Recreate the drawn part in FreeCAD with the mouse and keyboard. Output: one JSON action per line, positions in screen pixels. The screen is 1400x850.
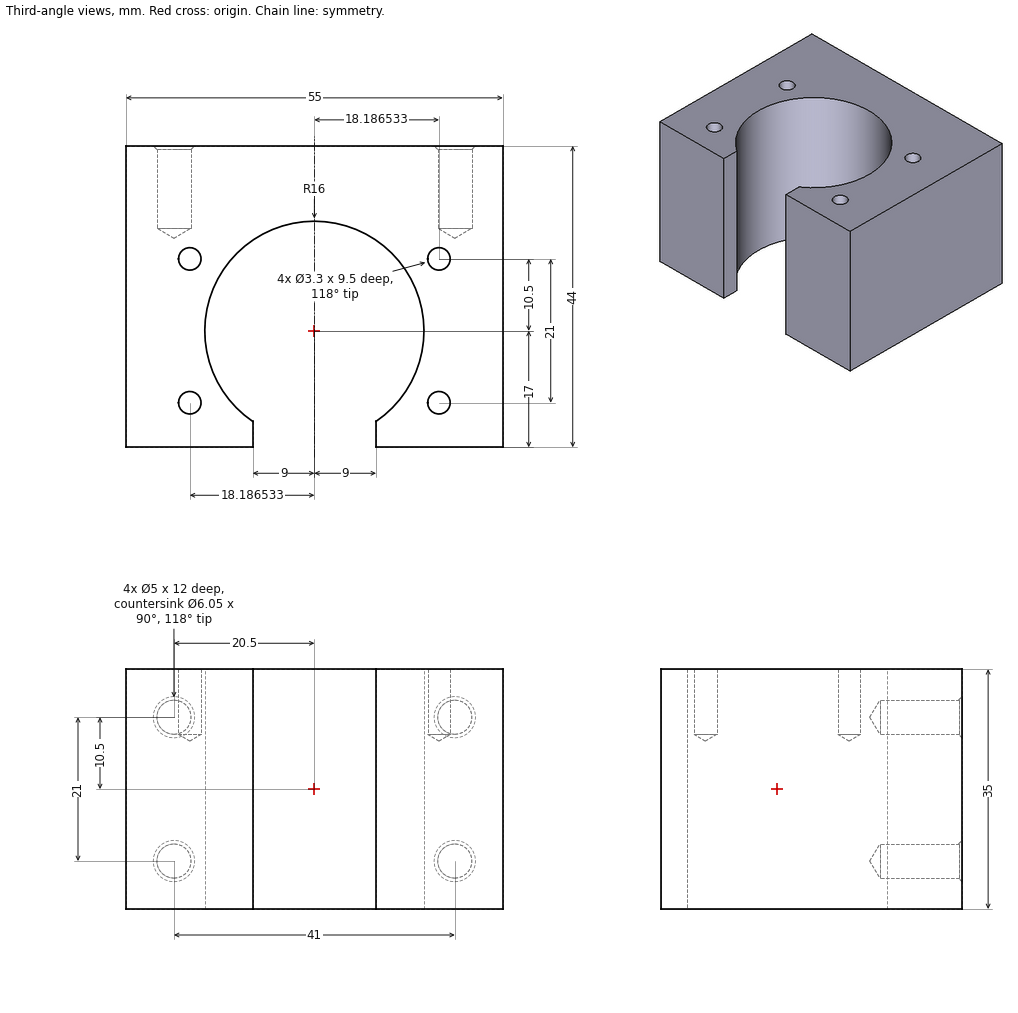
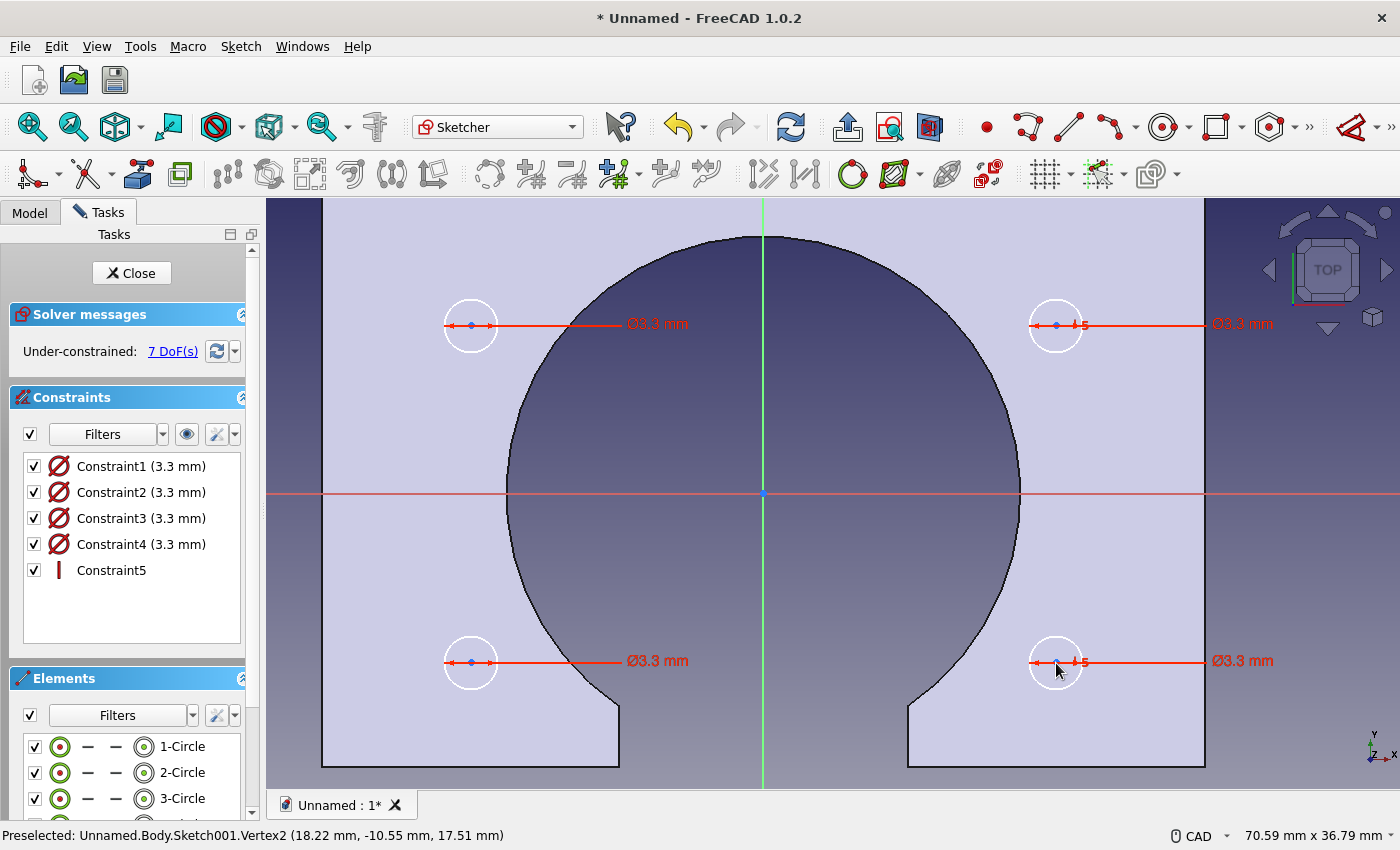
{"action": "left_click", "coordinate": [1056, 663]}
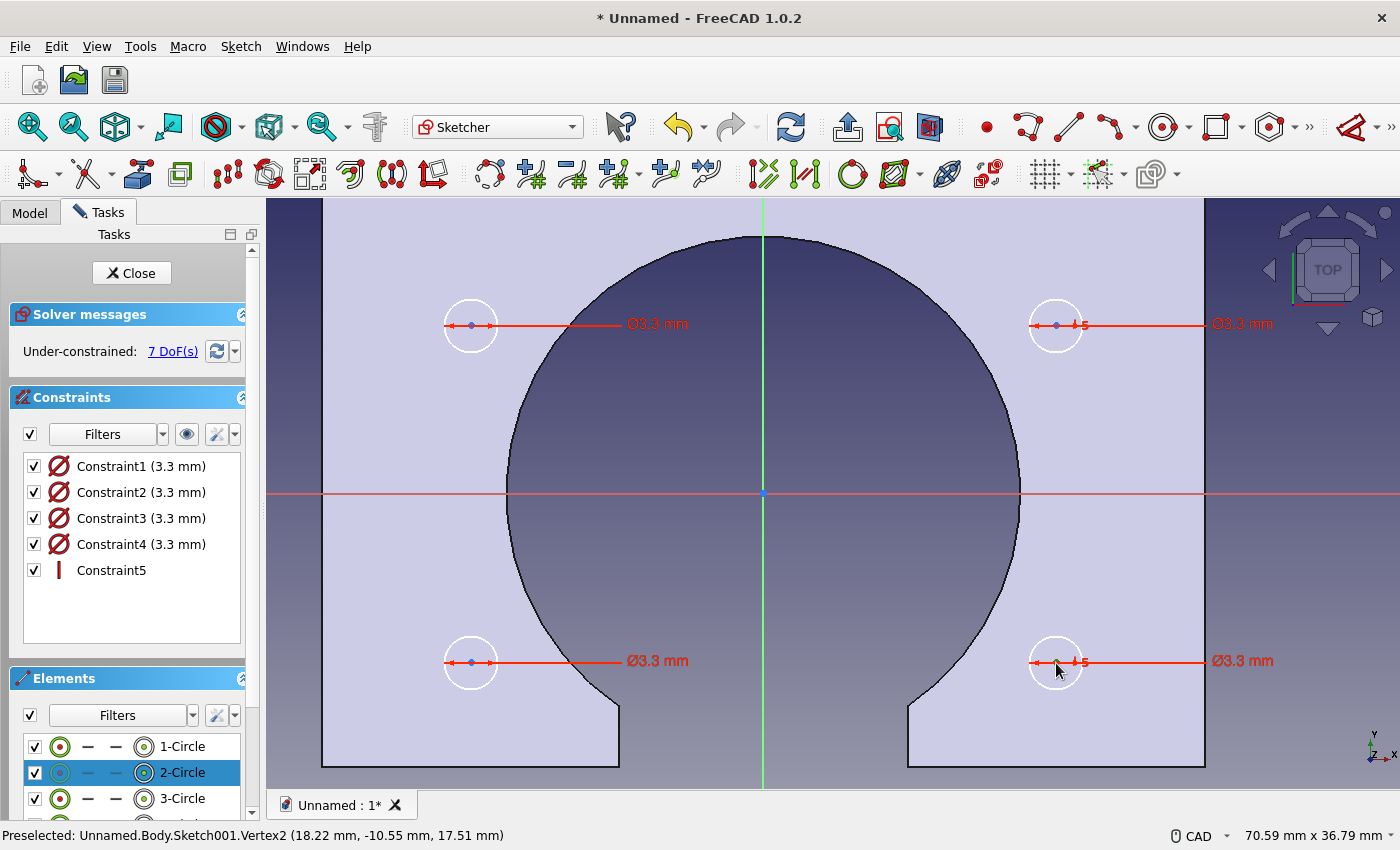
{"action": "left_click", "coordinate": [471, 663]}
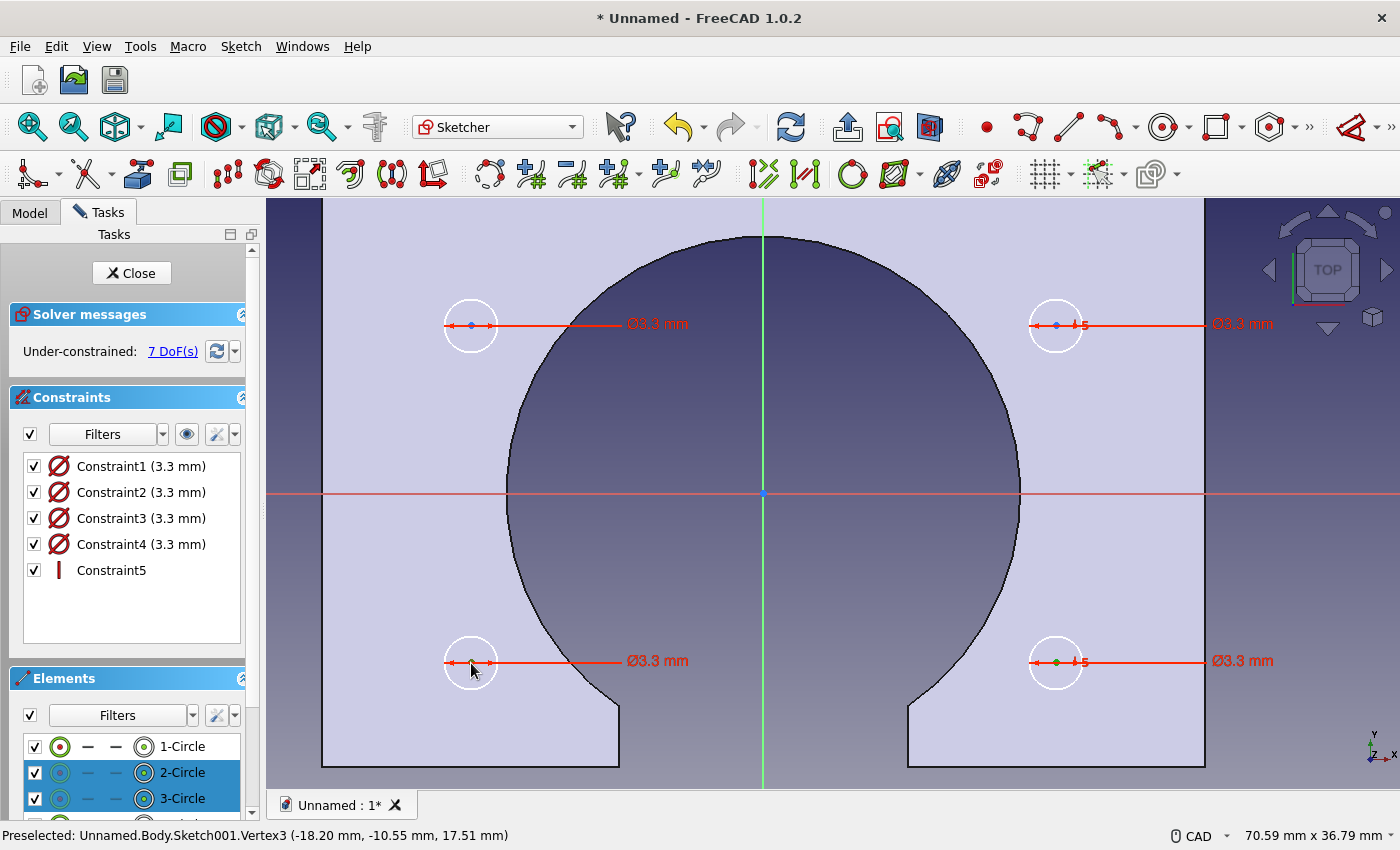
{"action": "key", "text": "h"}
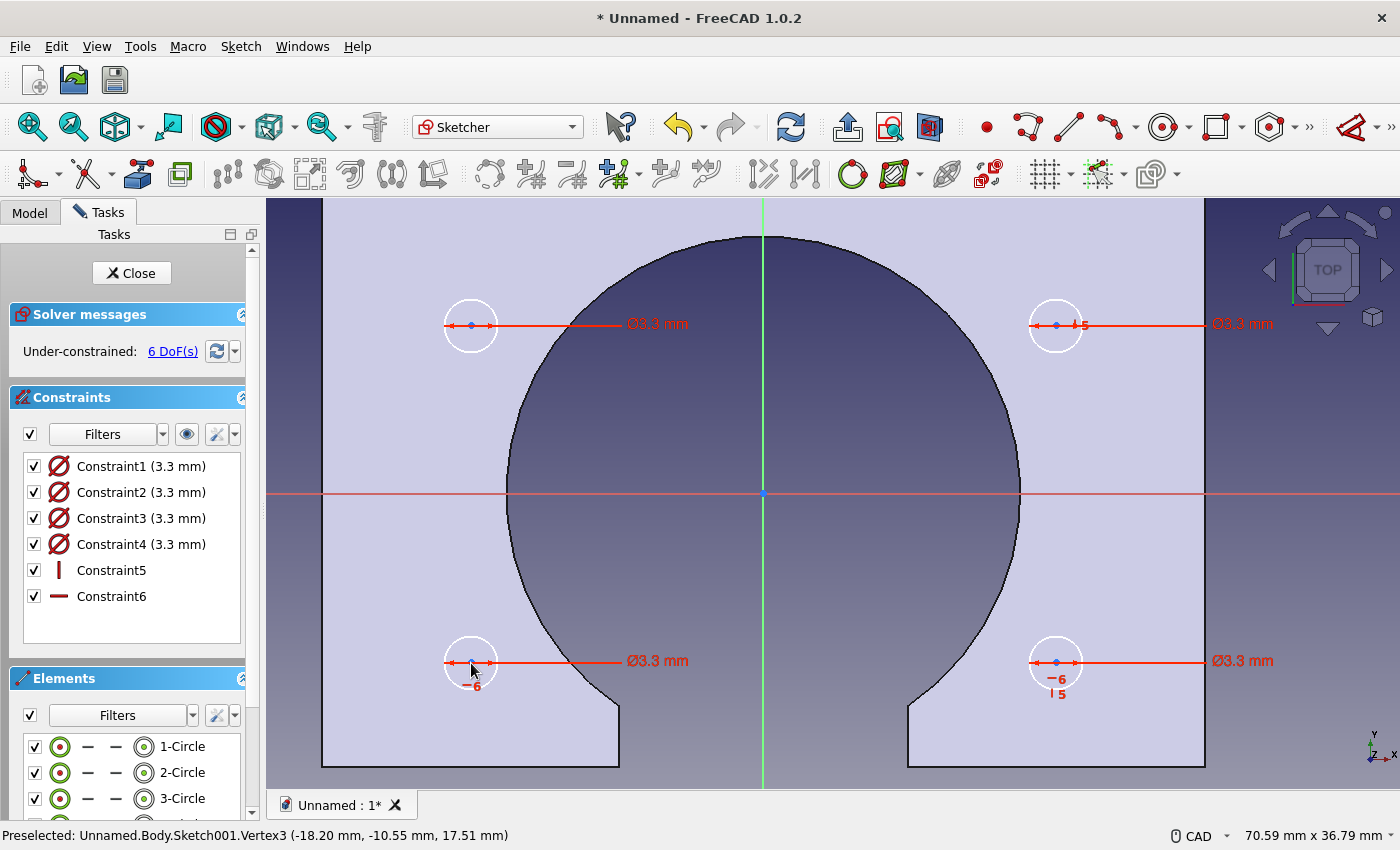
{"action": "left_click", "coordinate": [471, 663]}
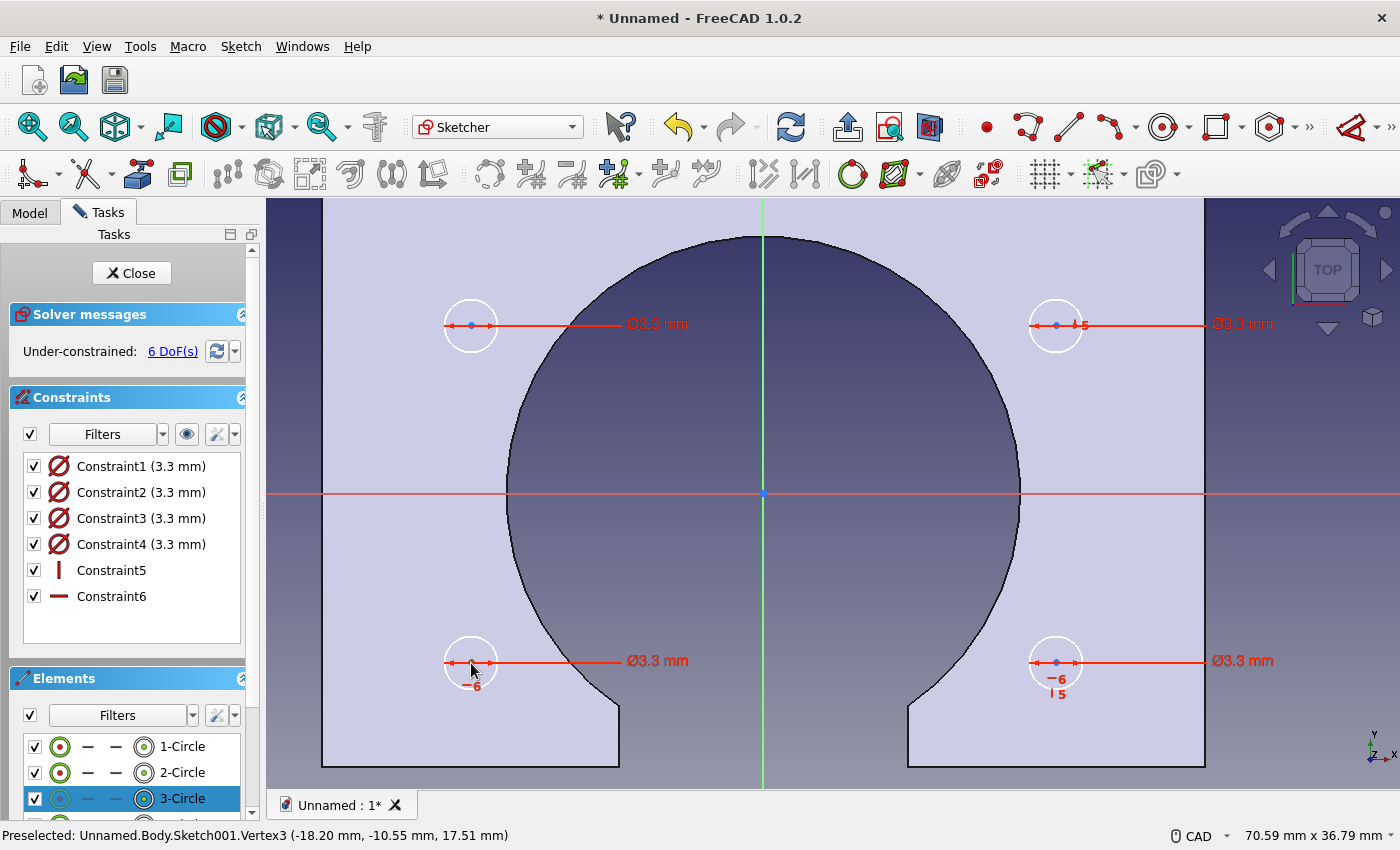
{"action": "left_click", "coordinate": [471, 326]}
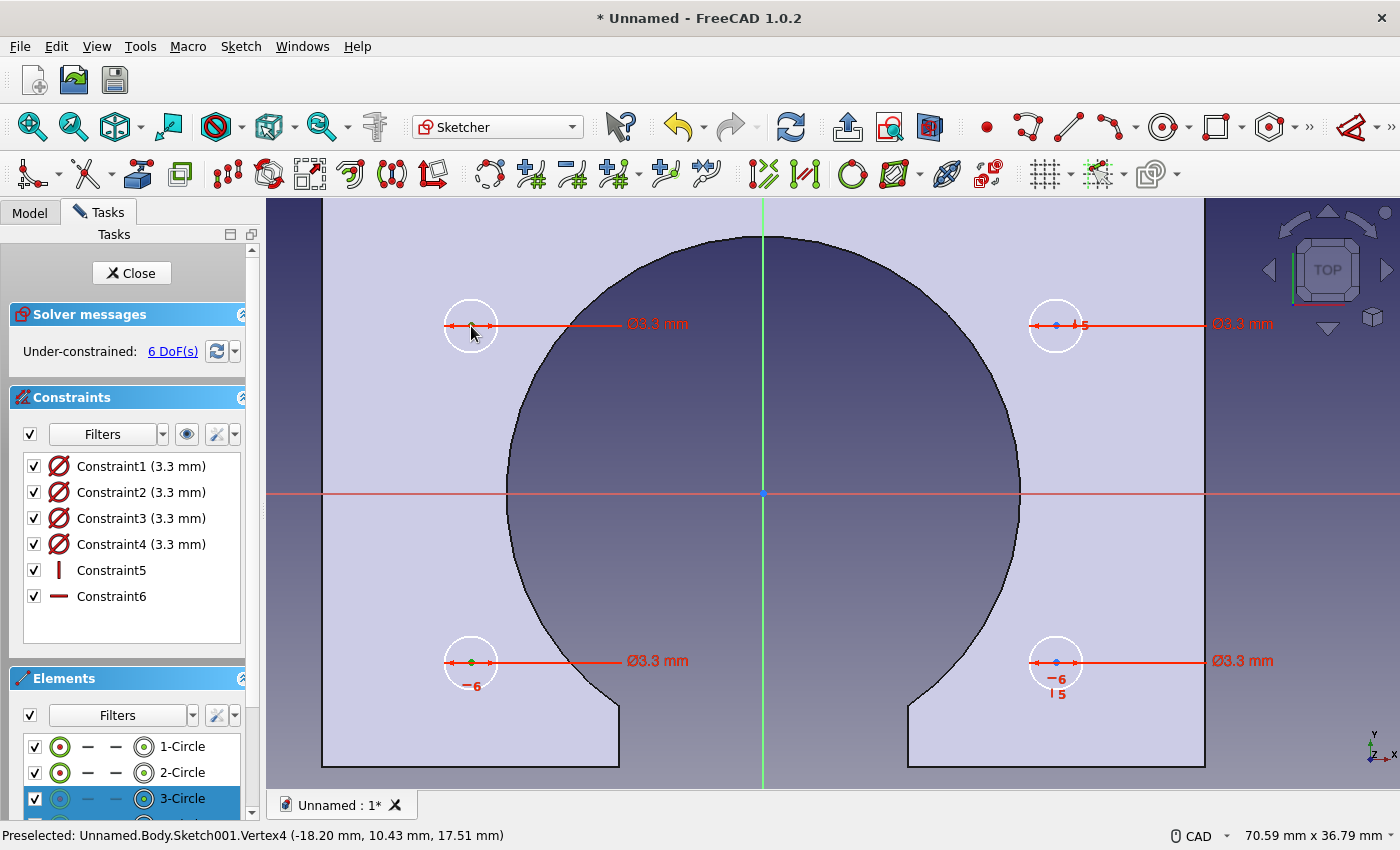
{"action": "key", "text": "v"}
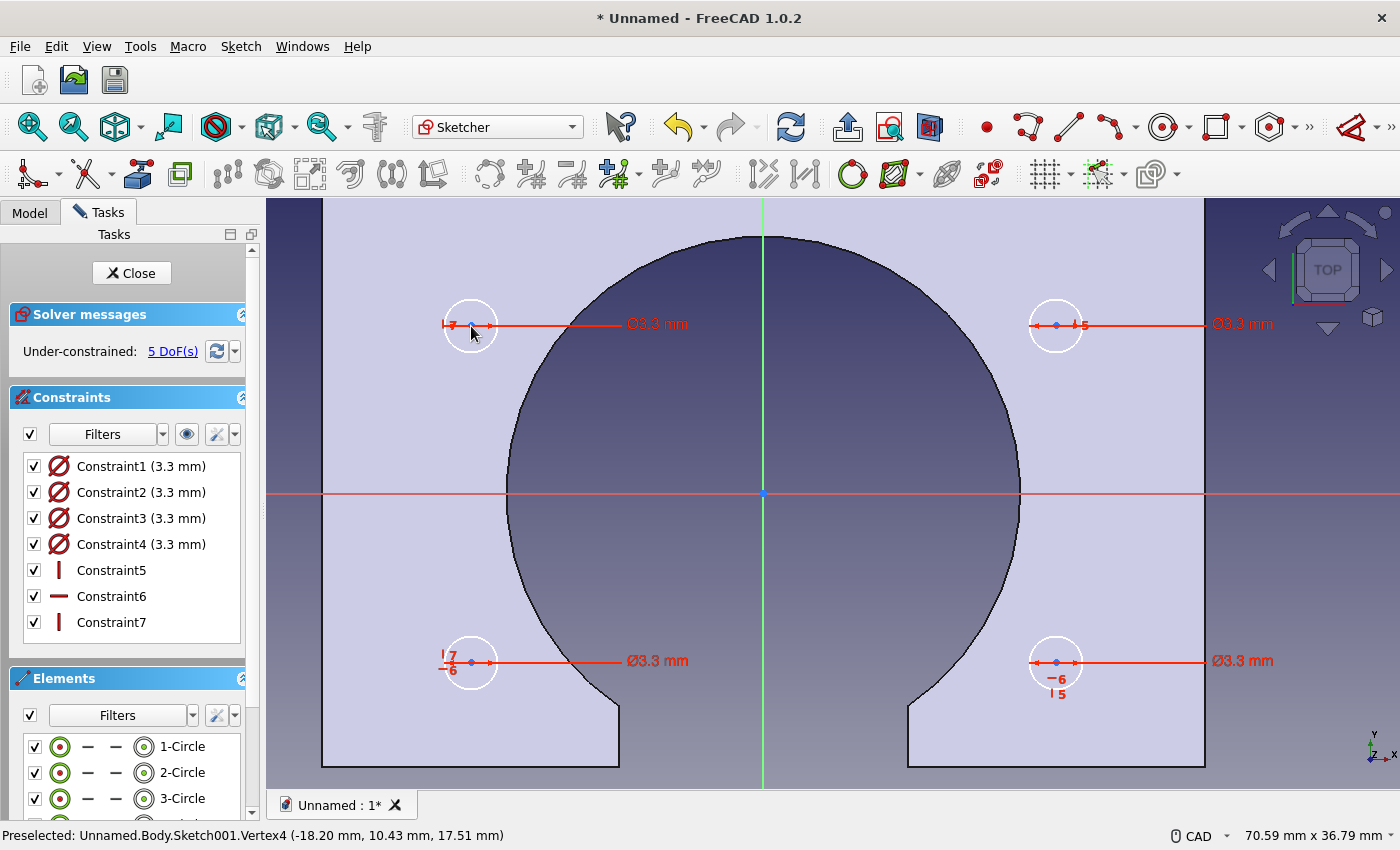
{"action": "left_click", "coordinate": [1056, 326]}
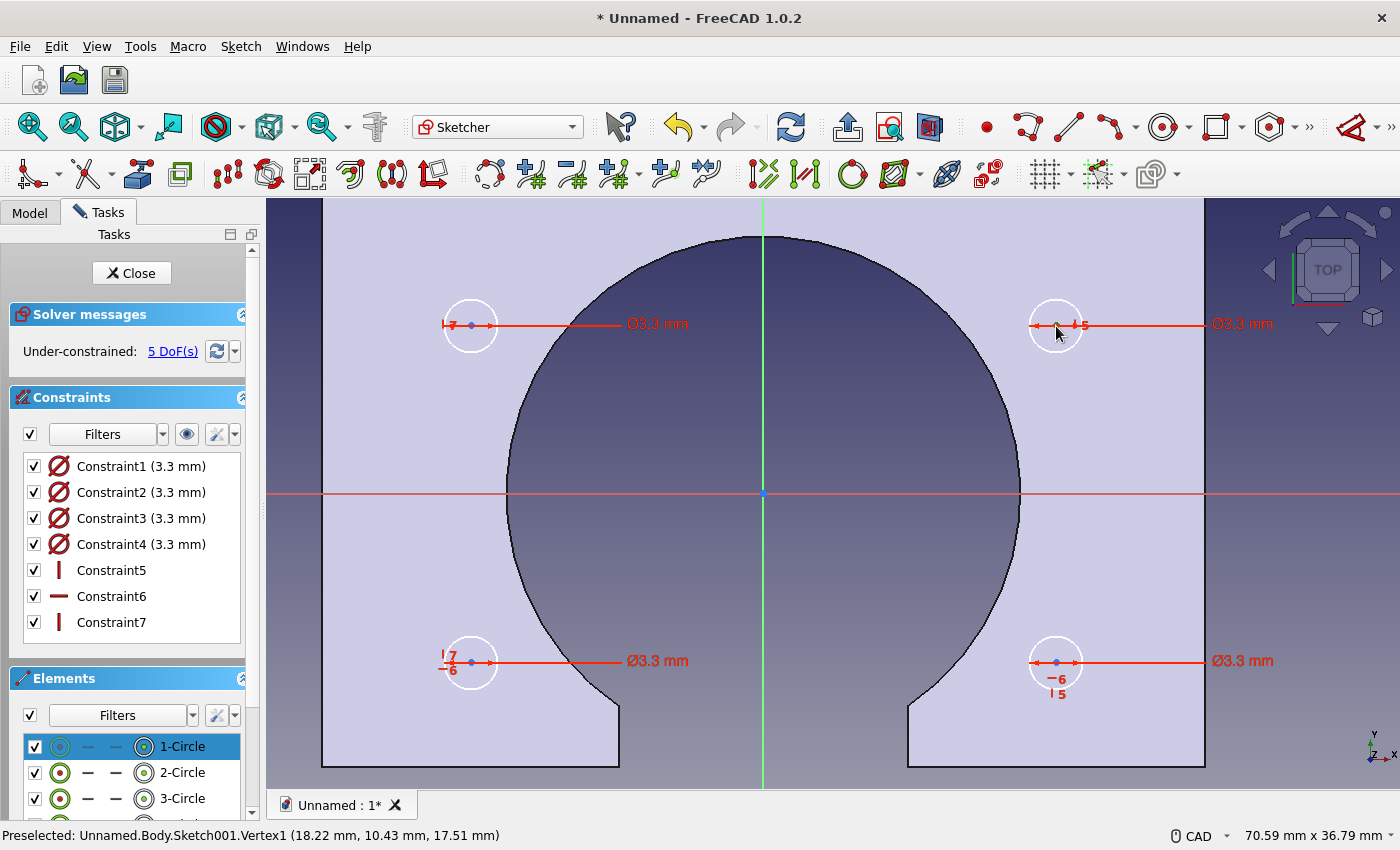
{"action": "left_click", "coordinate": [471, 326]}